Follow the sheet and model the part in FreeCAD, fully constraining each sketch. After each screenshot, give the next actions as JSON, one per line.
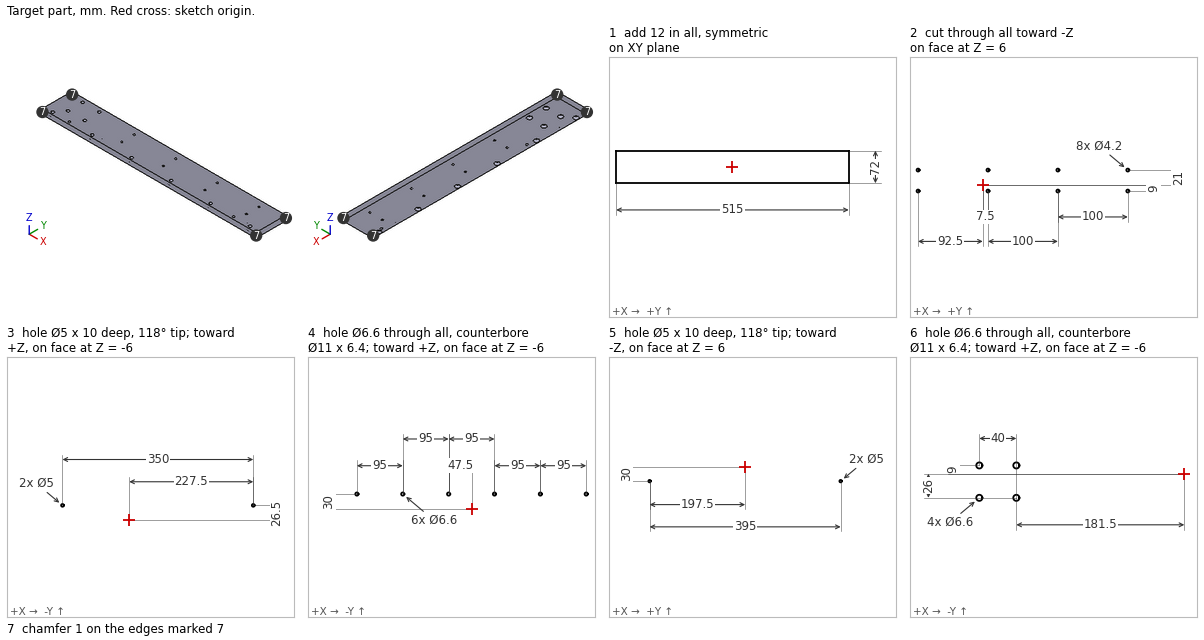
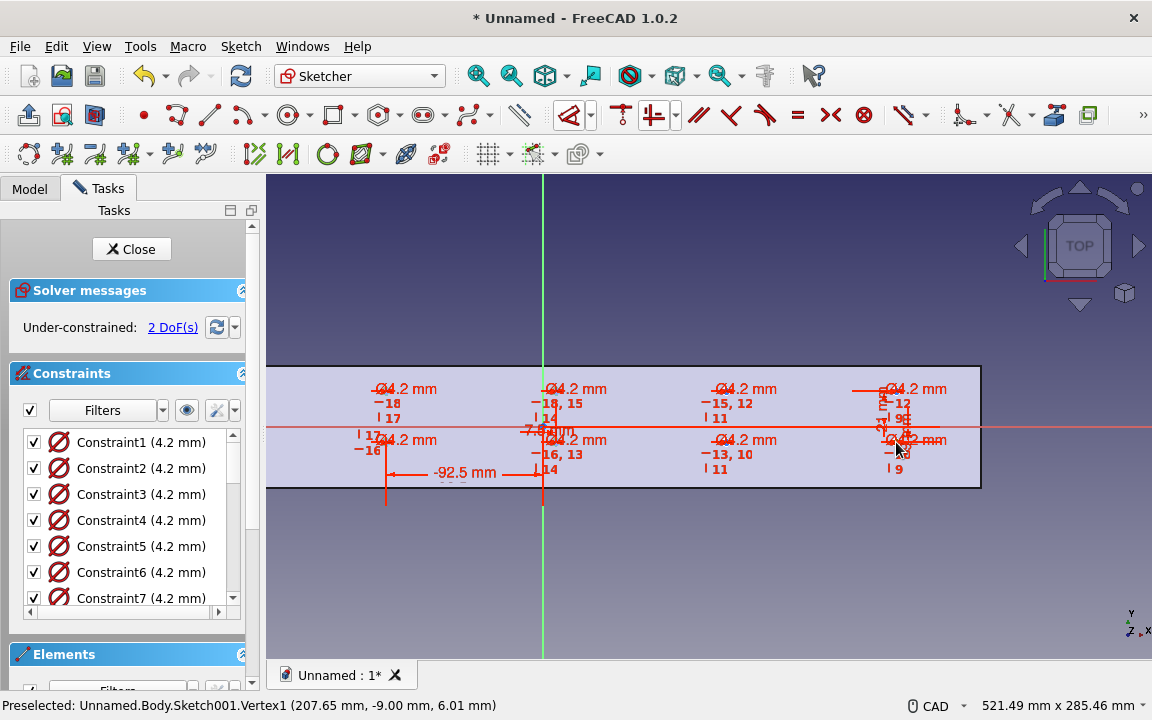
{"action": "left_click", "coordinate": [726, 442]}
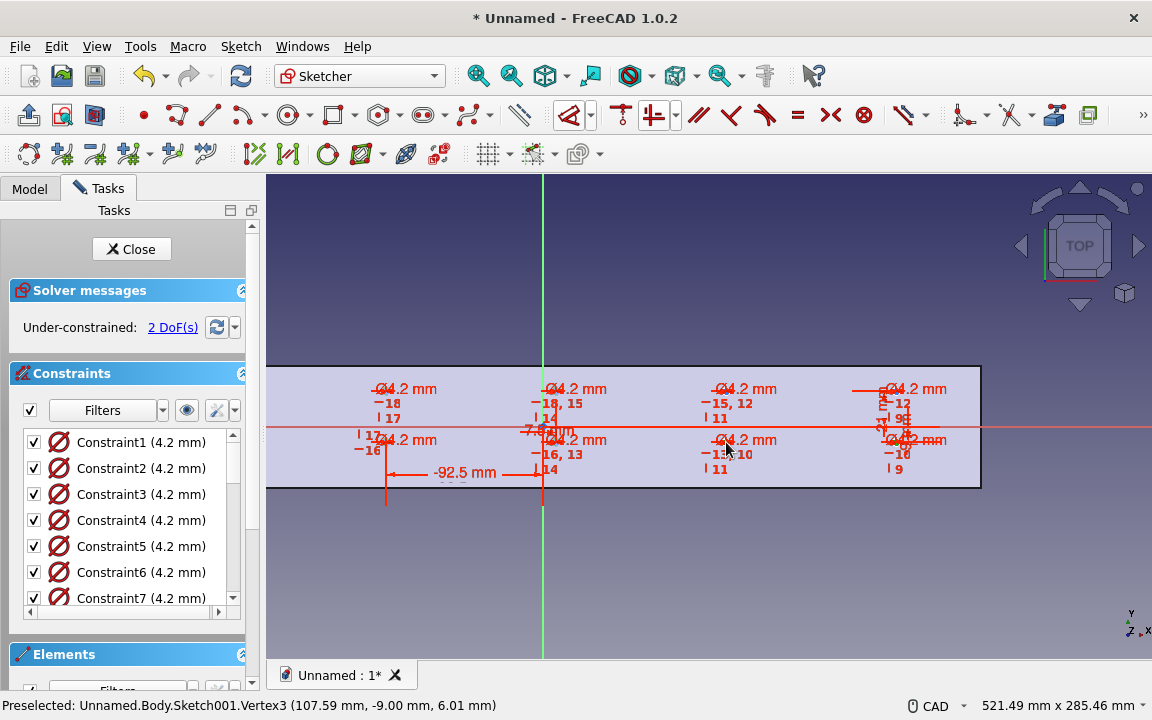
{"action": "key", "text": "l"}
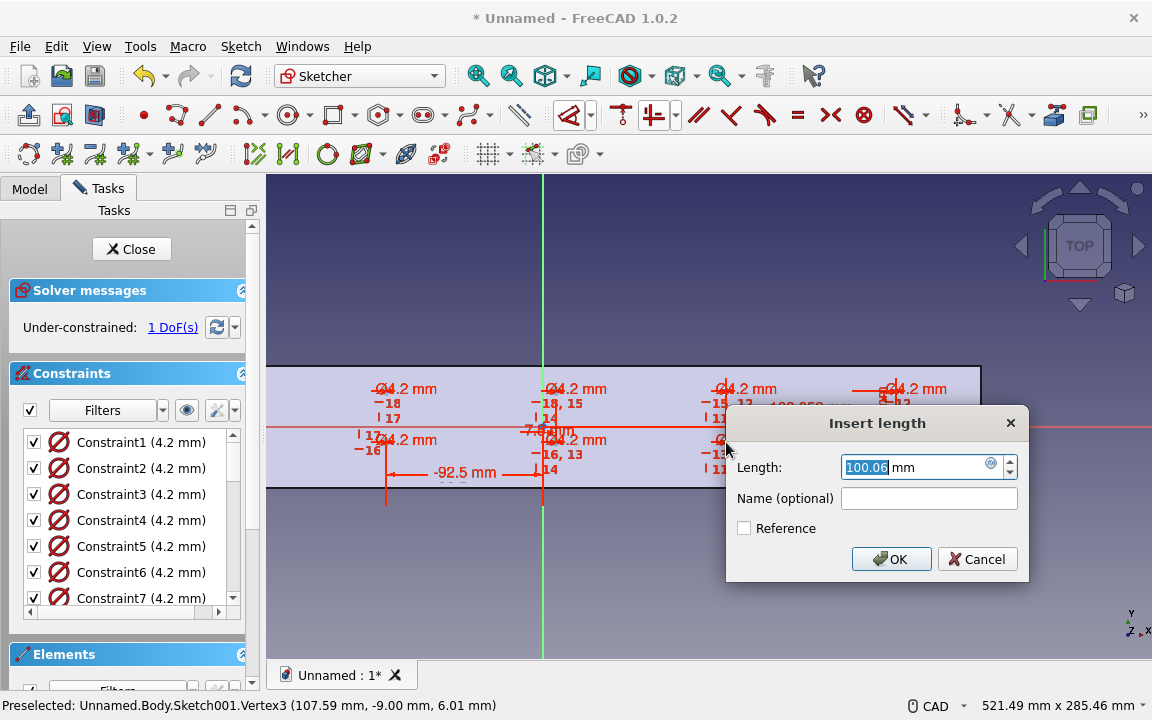
{"action": "type", "text": "100"}
{"action": "key", "text": "Return"}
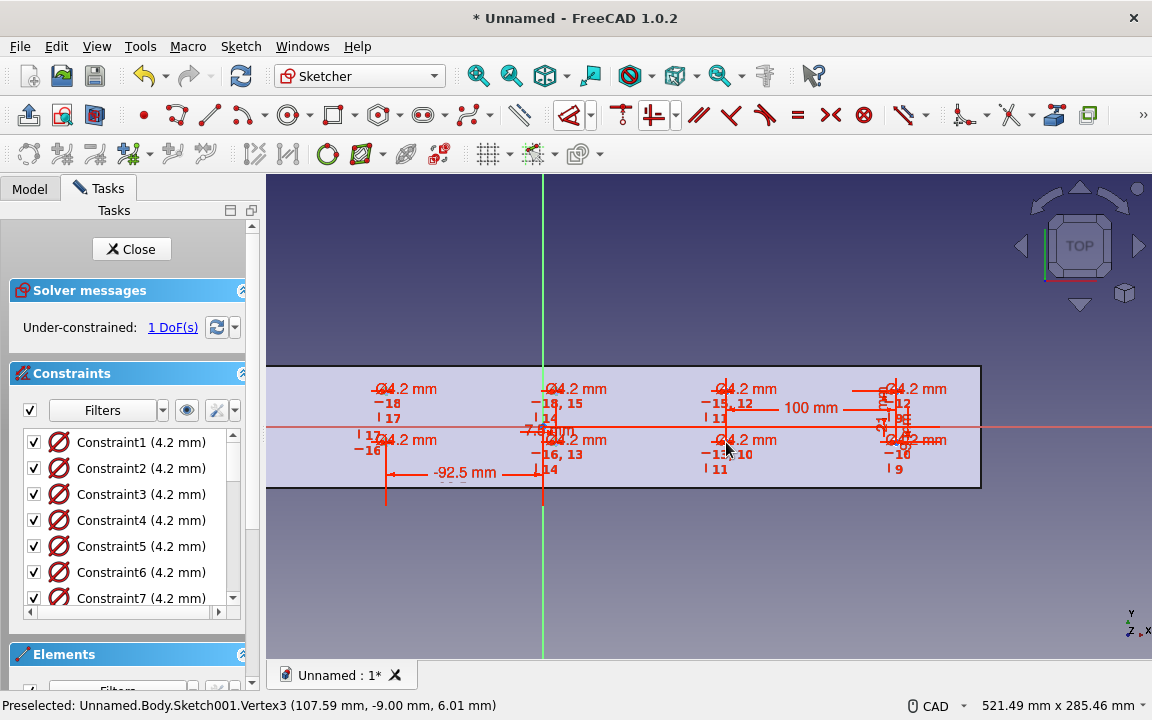
{"action": "left_click", "coordinate": [726, 442]}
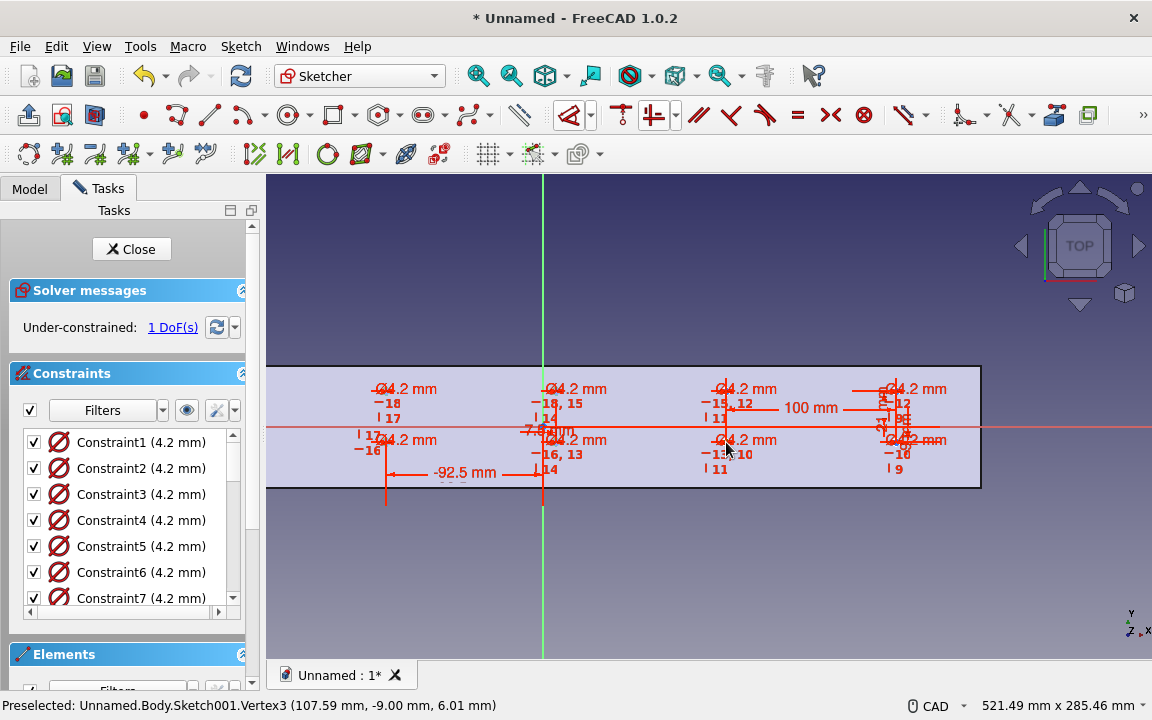
{"action": "left_click", "coordinate": [556, 442]}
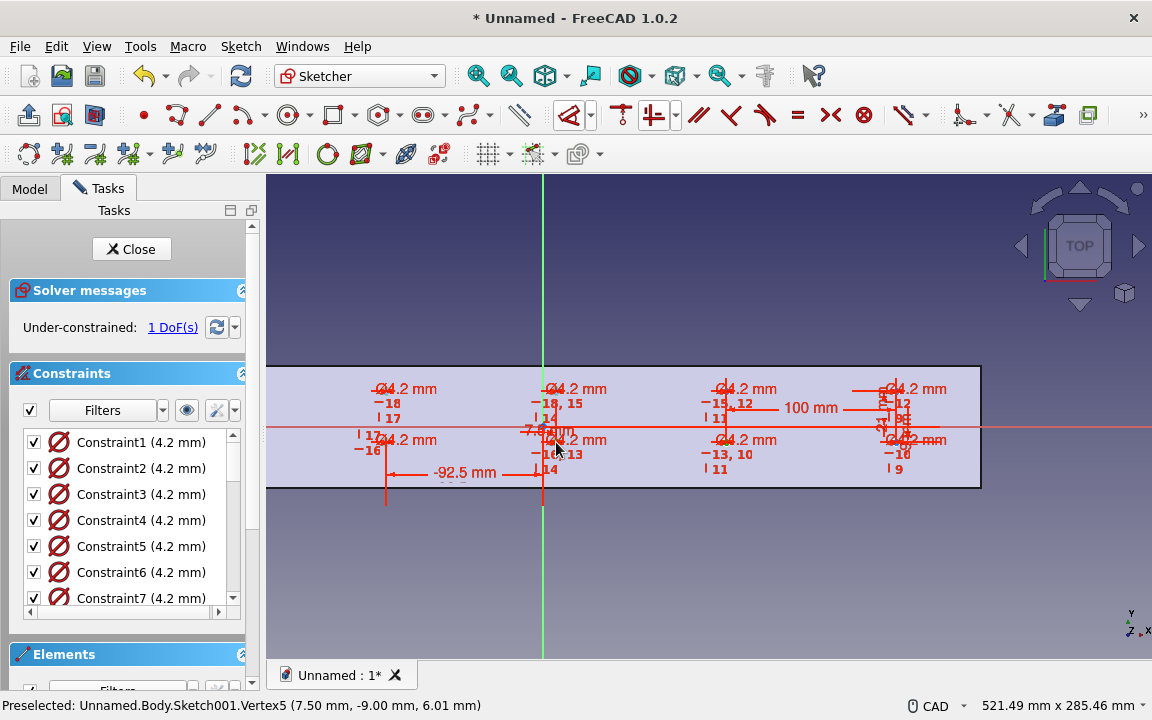
{"action": "left_click", "coordinate": [590, 116]}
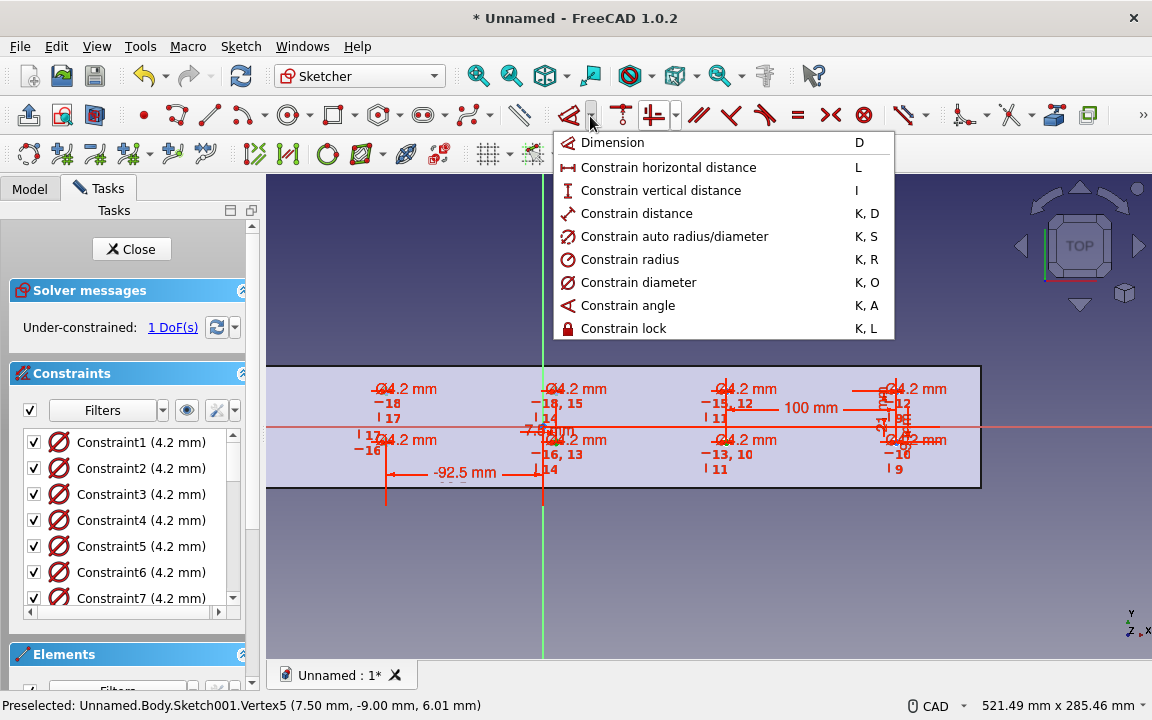
{"action": "left_click", "coordinate": [724, 168]}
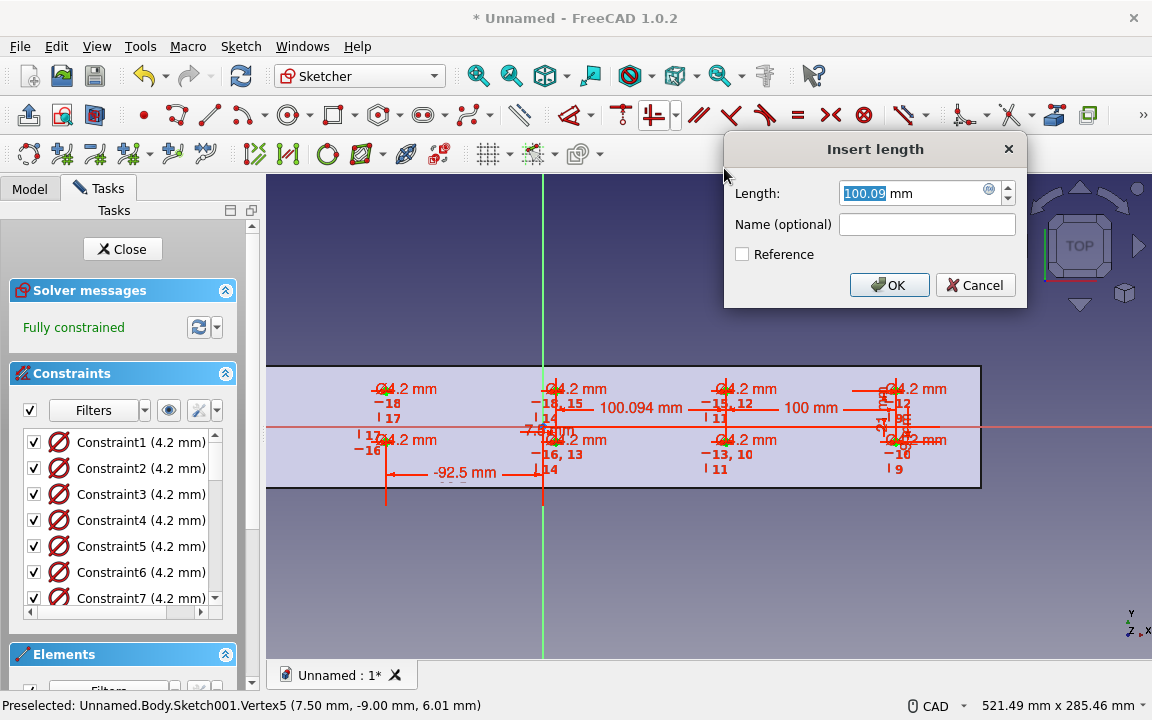
{"action": "type", "text": "100"}
{"action": "key", "text": "Return"}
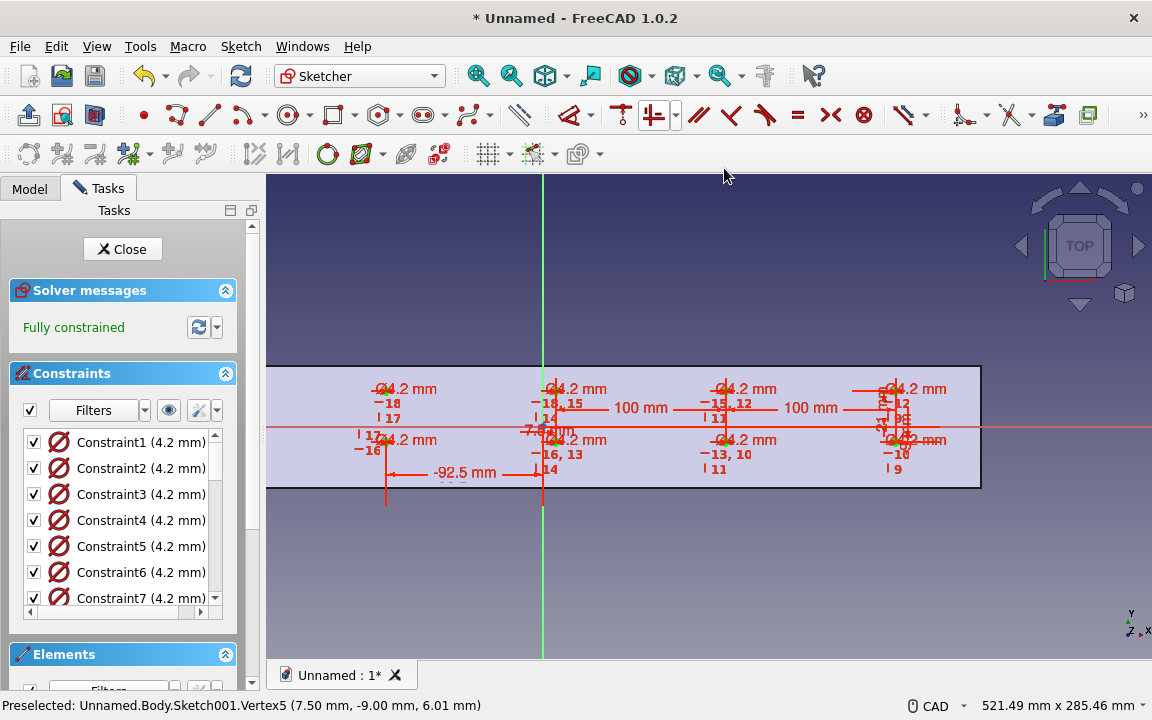
{"action": "left_click", "coordinate": [123, 249]}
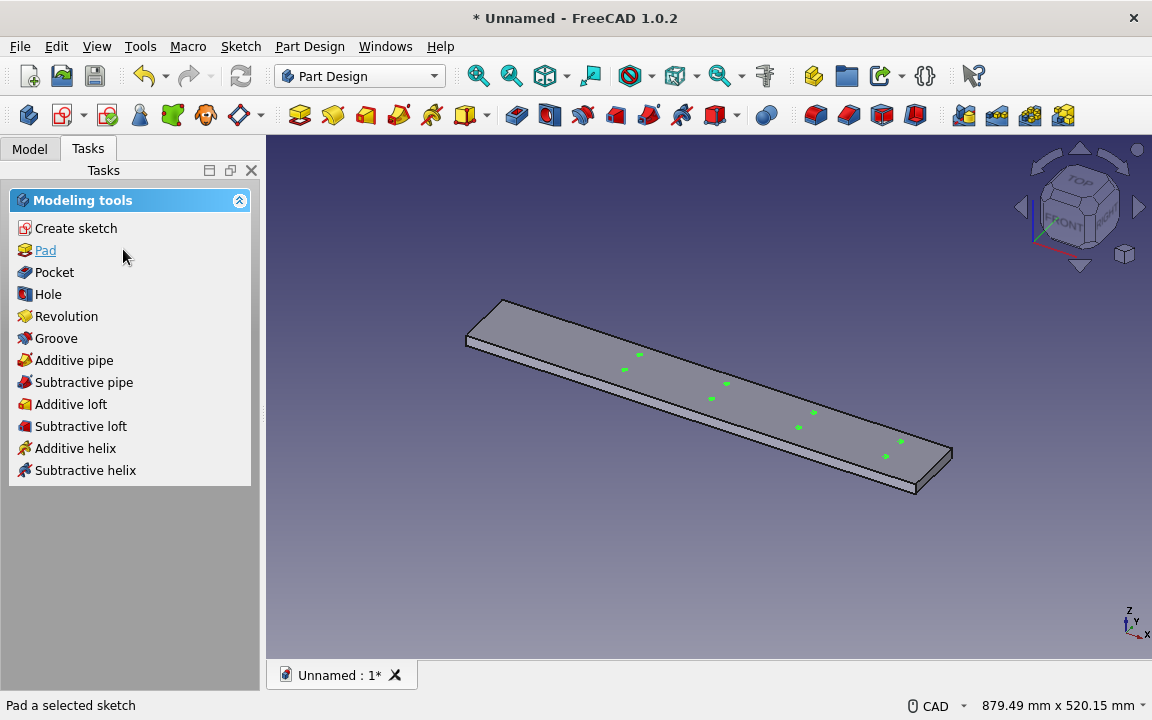
{"action": "left_click", "coordinate": [517, 116]}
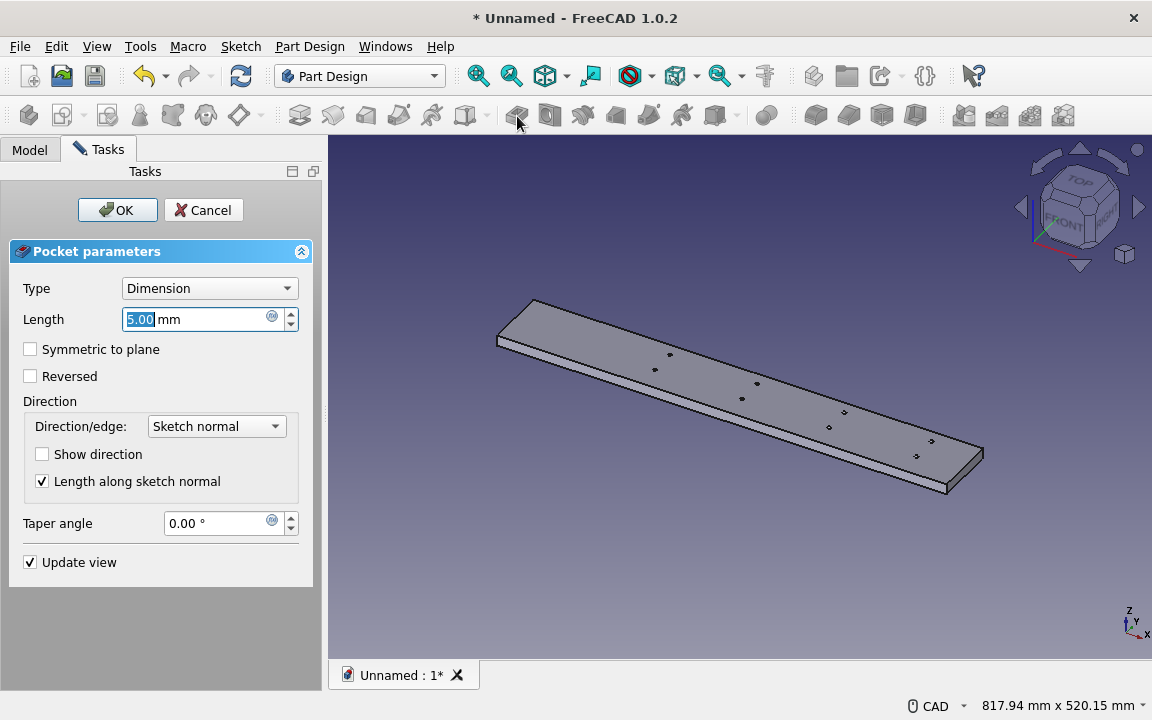
{"action": "left_click", "coordinate": [210, 288]}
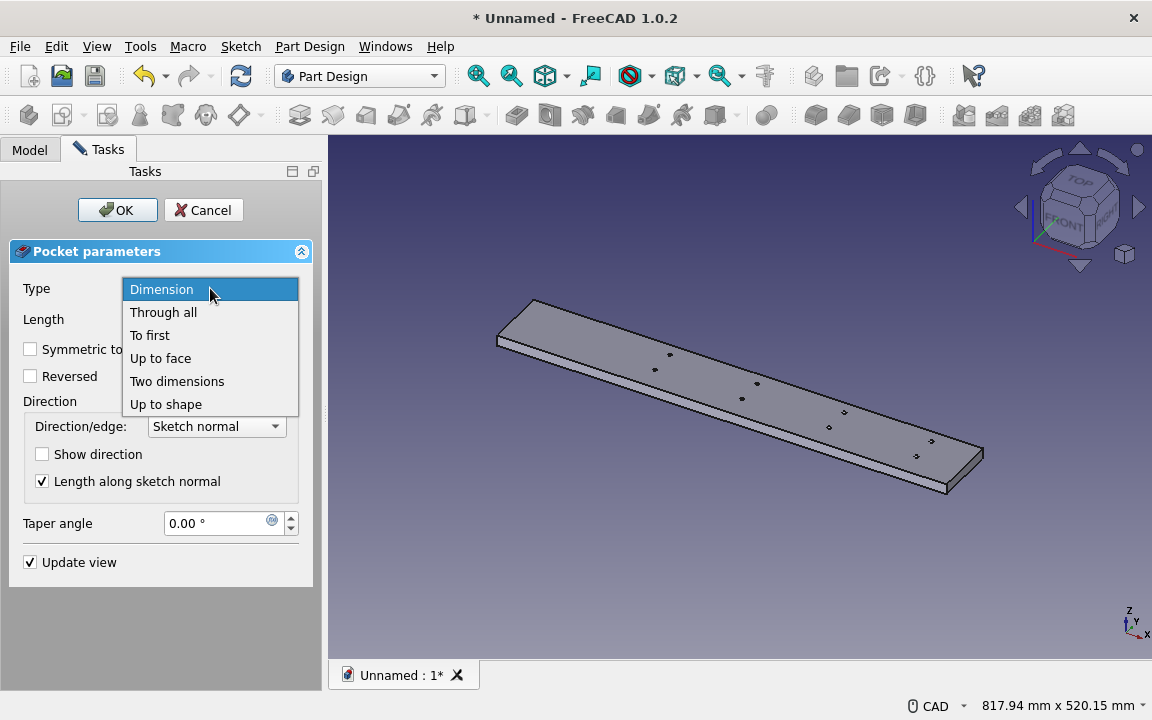
{"action": "left_click", "coordinate": [208, 312]}